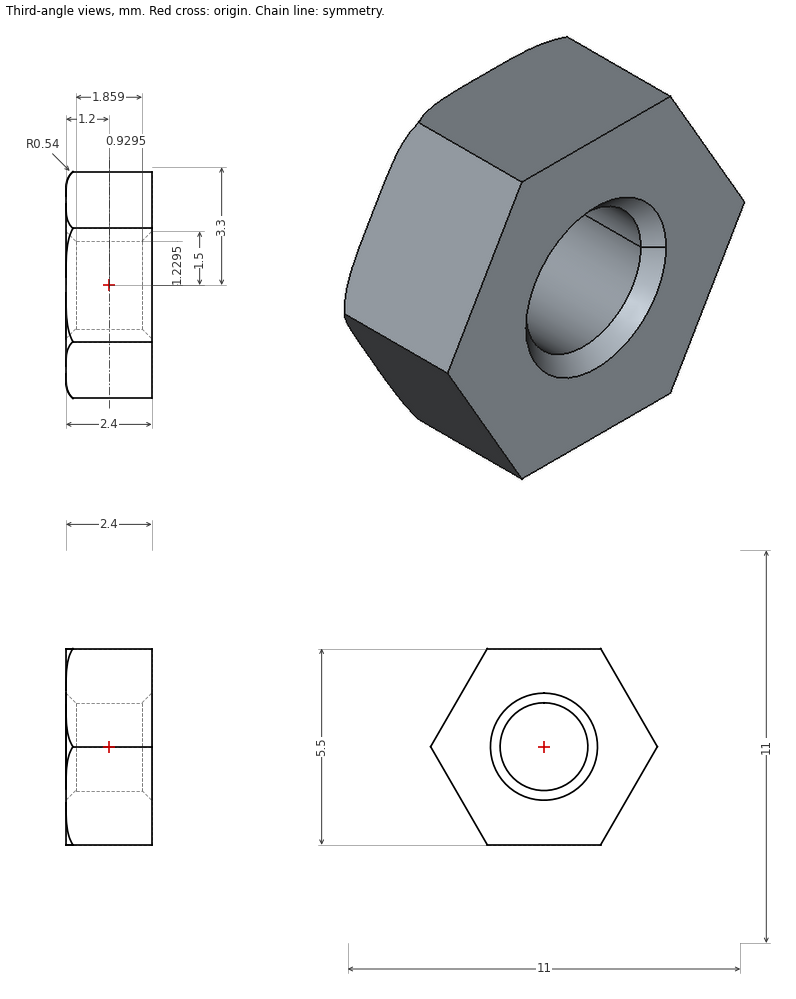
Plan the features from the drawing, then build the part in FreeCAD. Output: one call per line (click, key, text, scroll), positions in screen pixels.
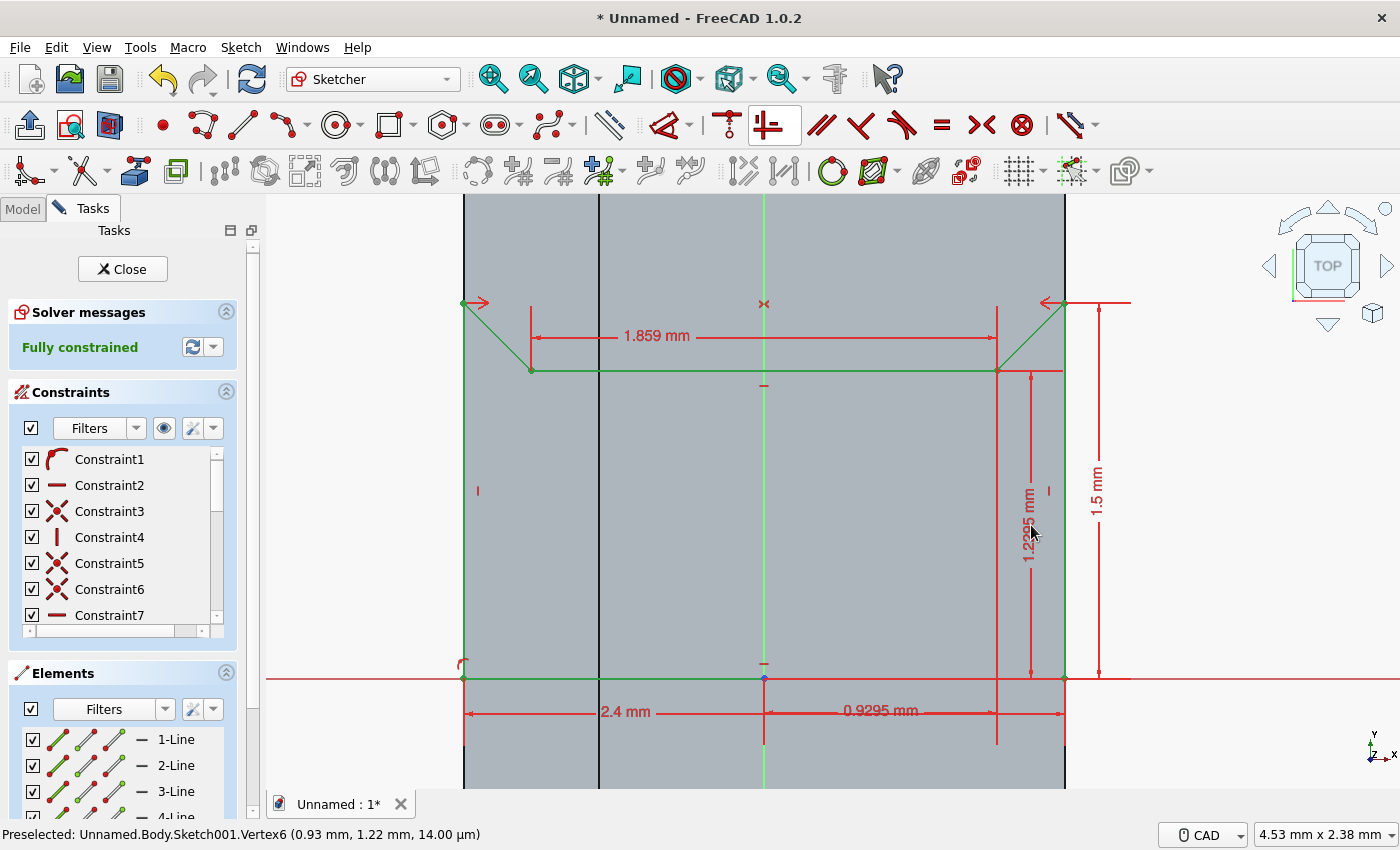
click(123, 269)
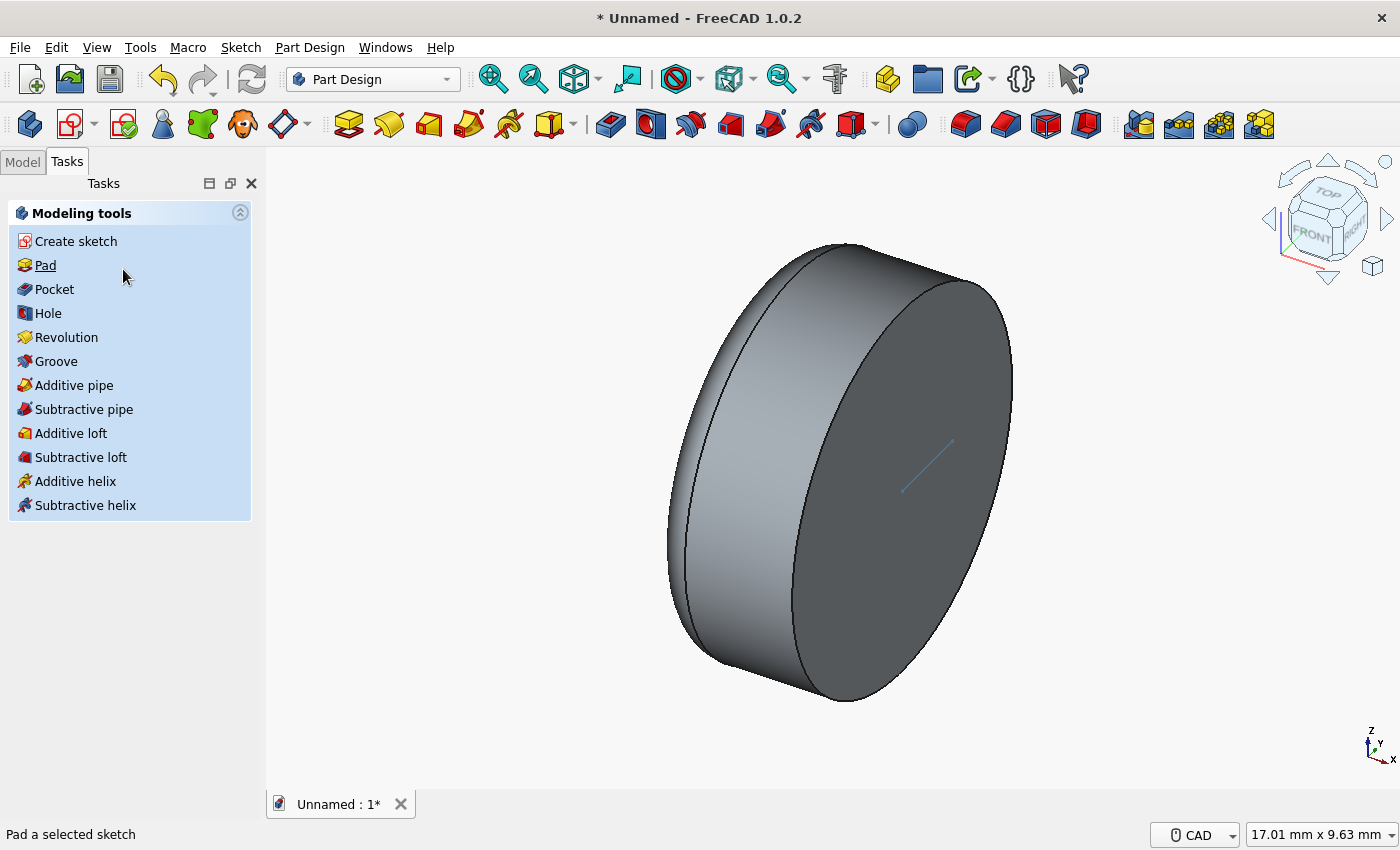
click(692, 124)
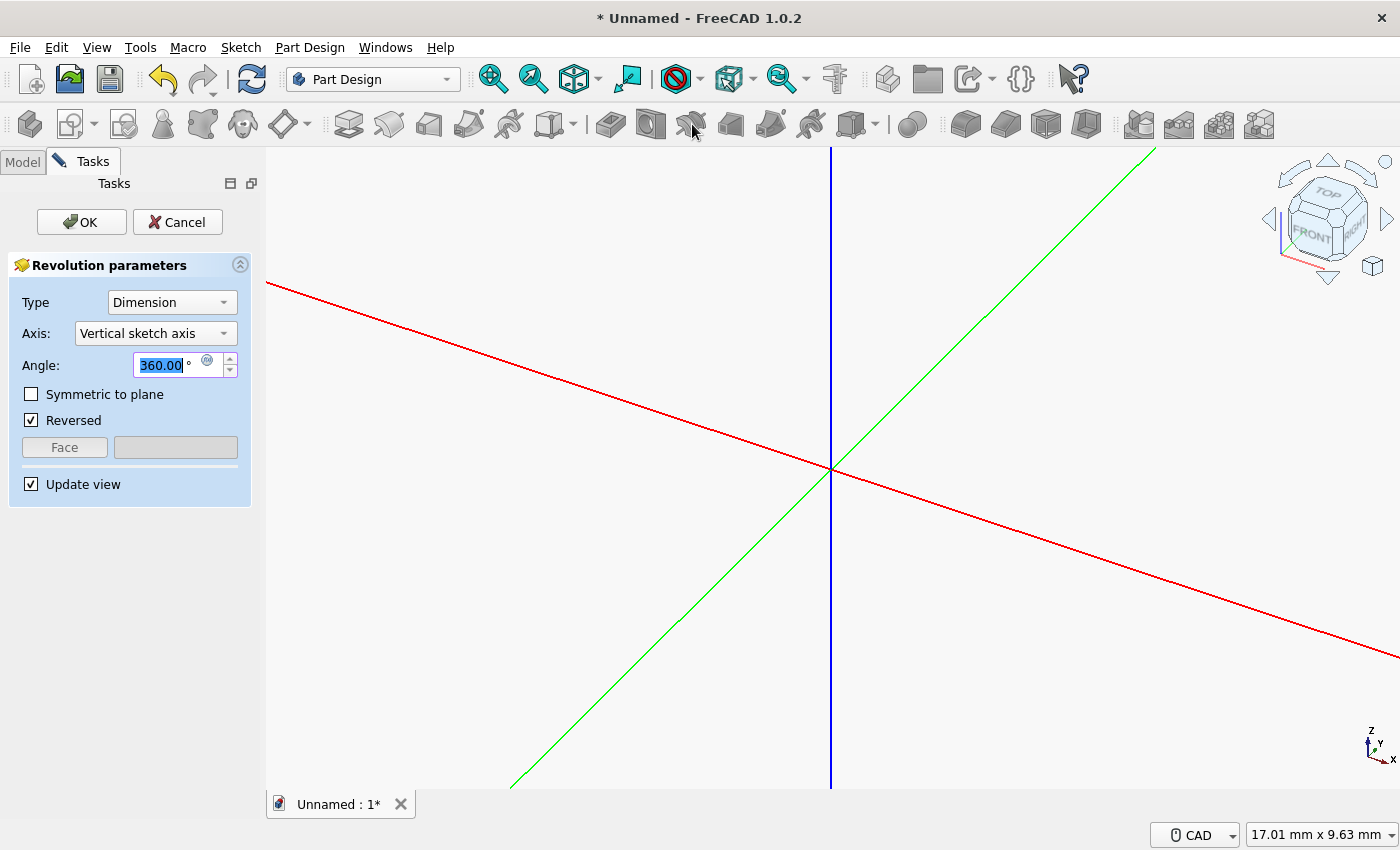
click(156, 334)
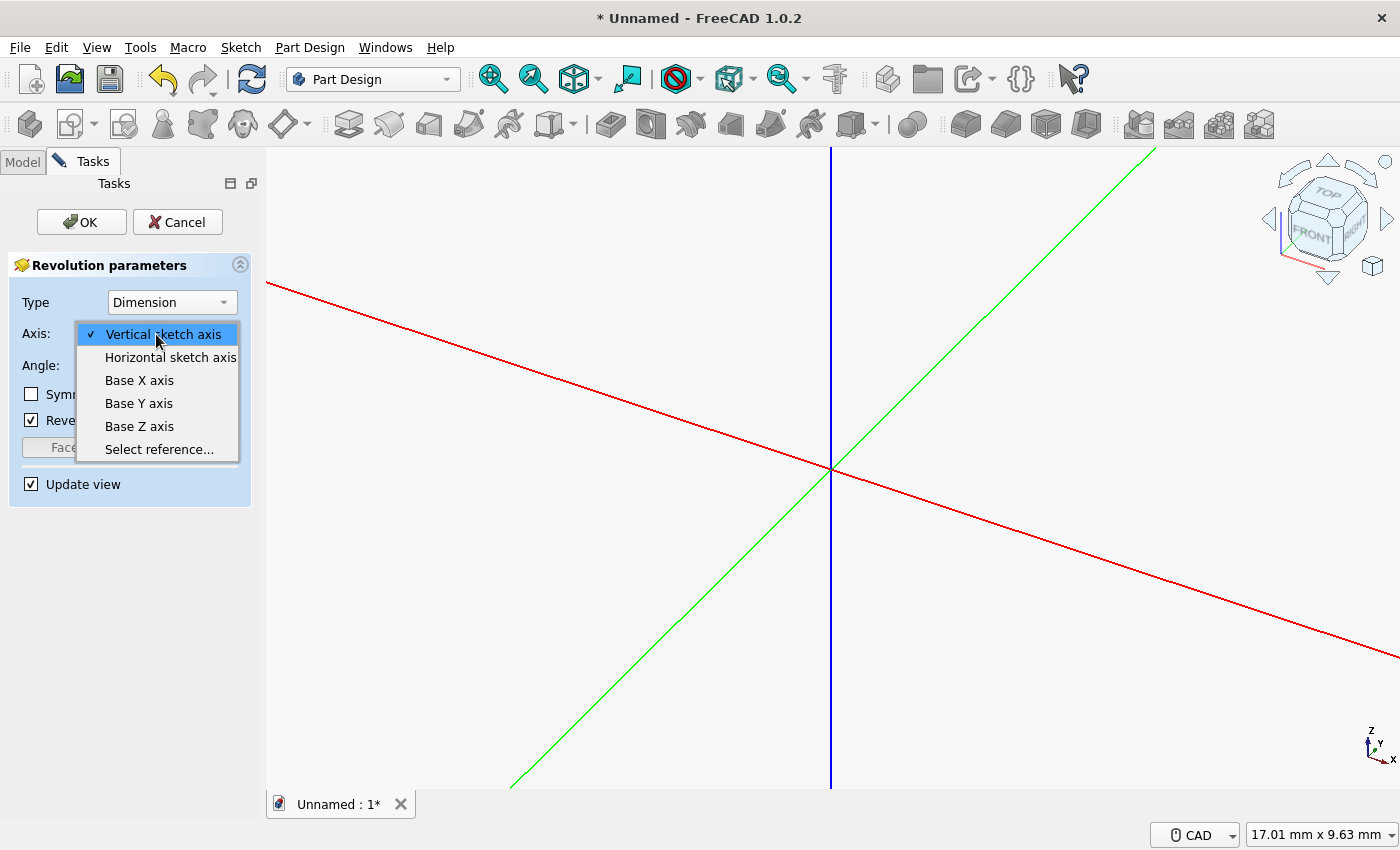
click(156, 358)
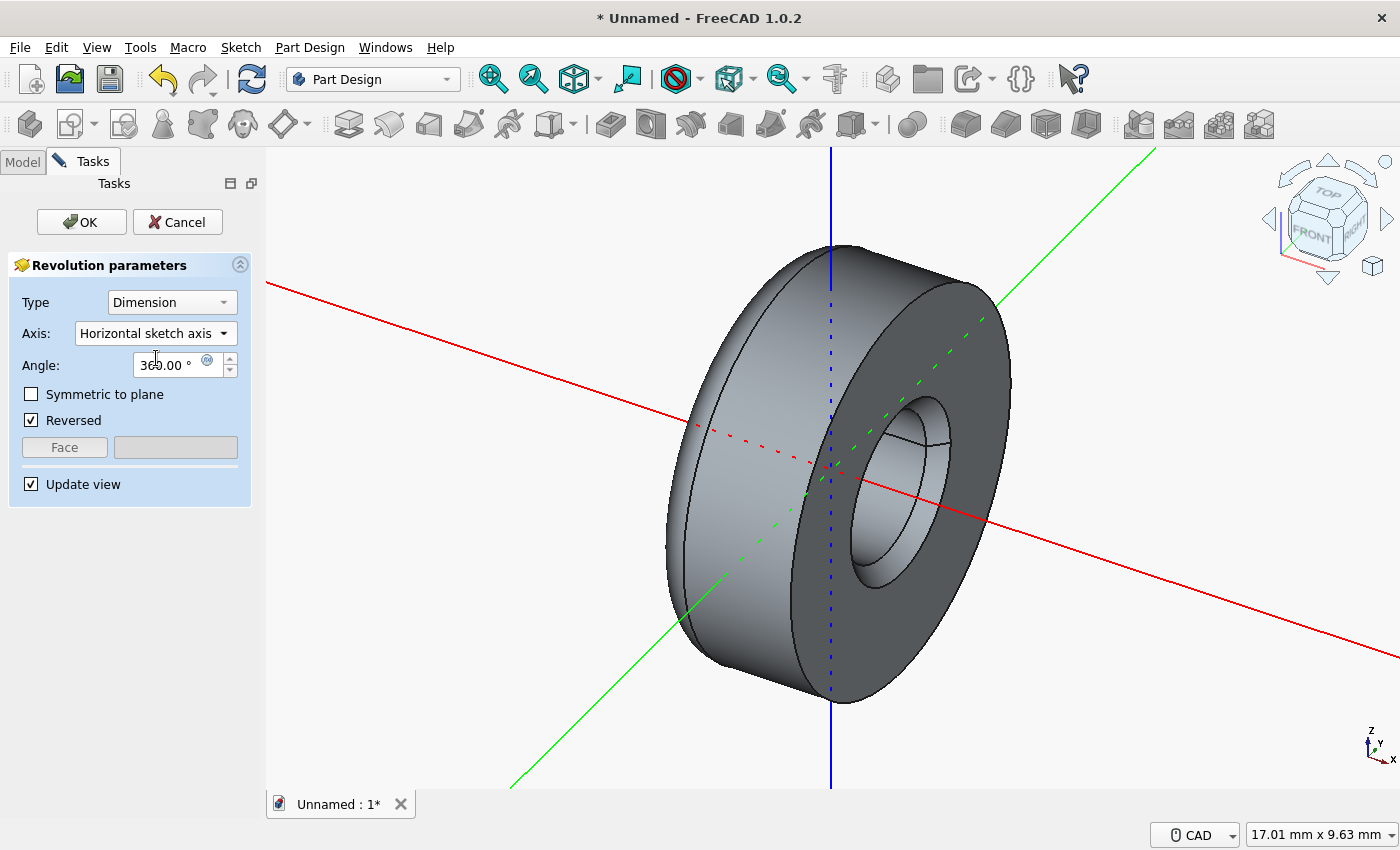
click(82, 222)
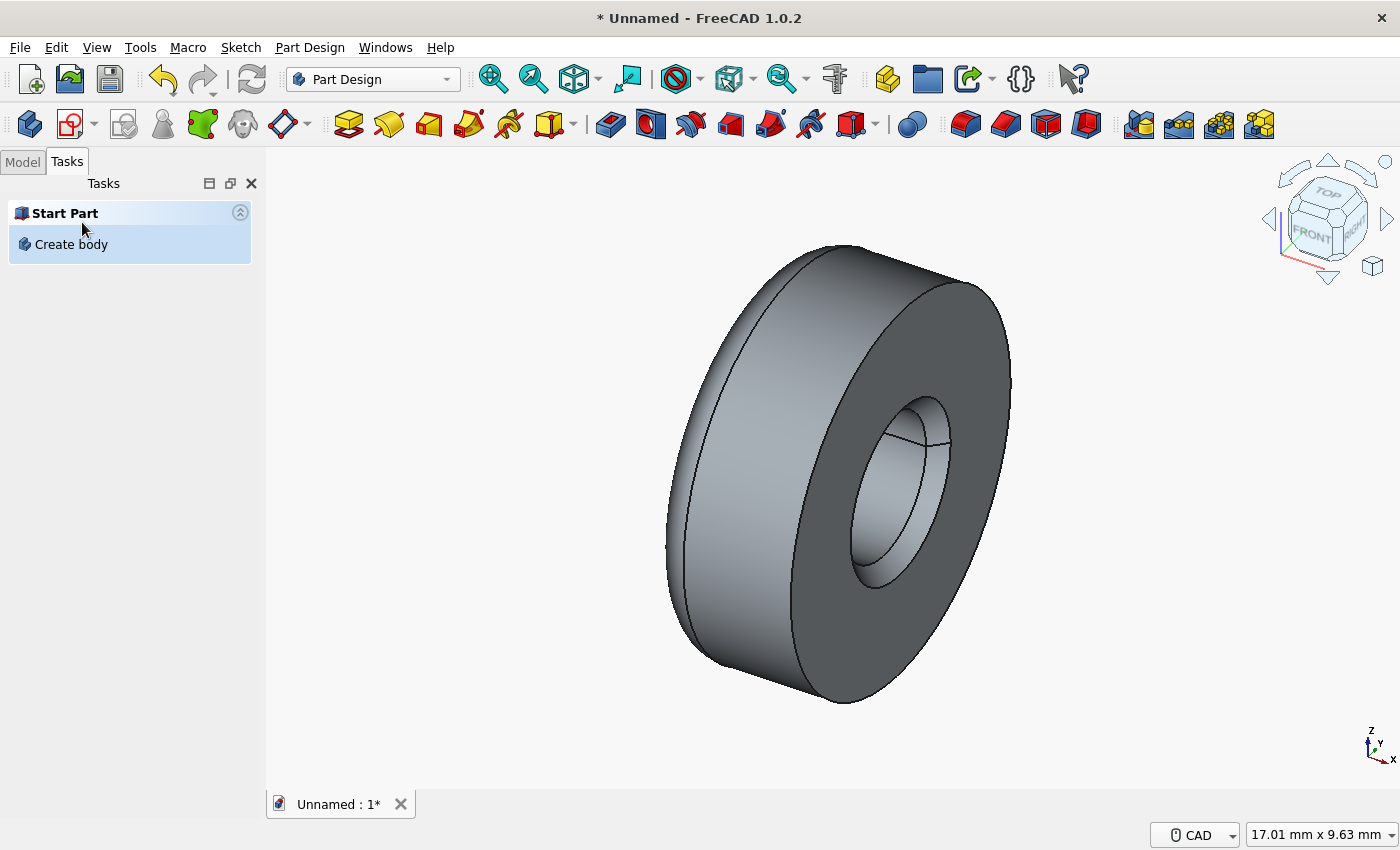
click(70, 124)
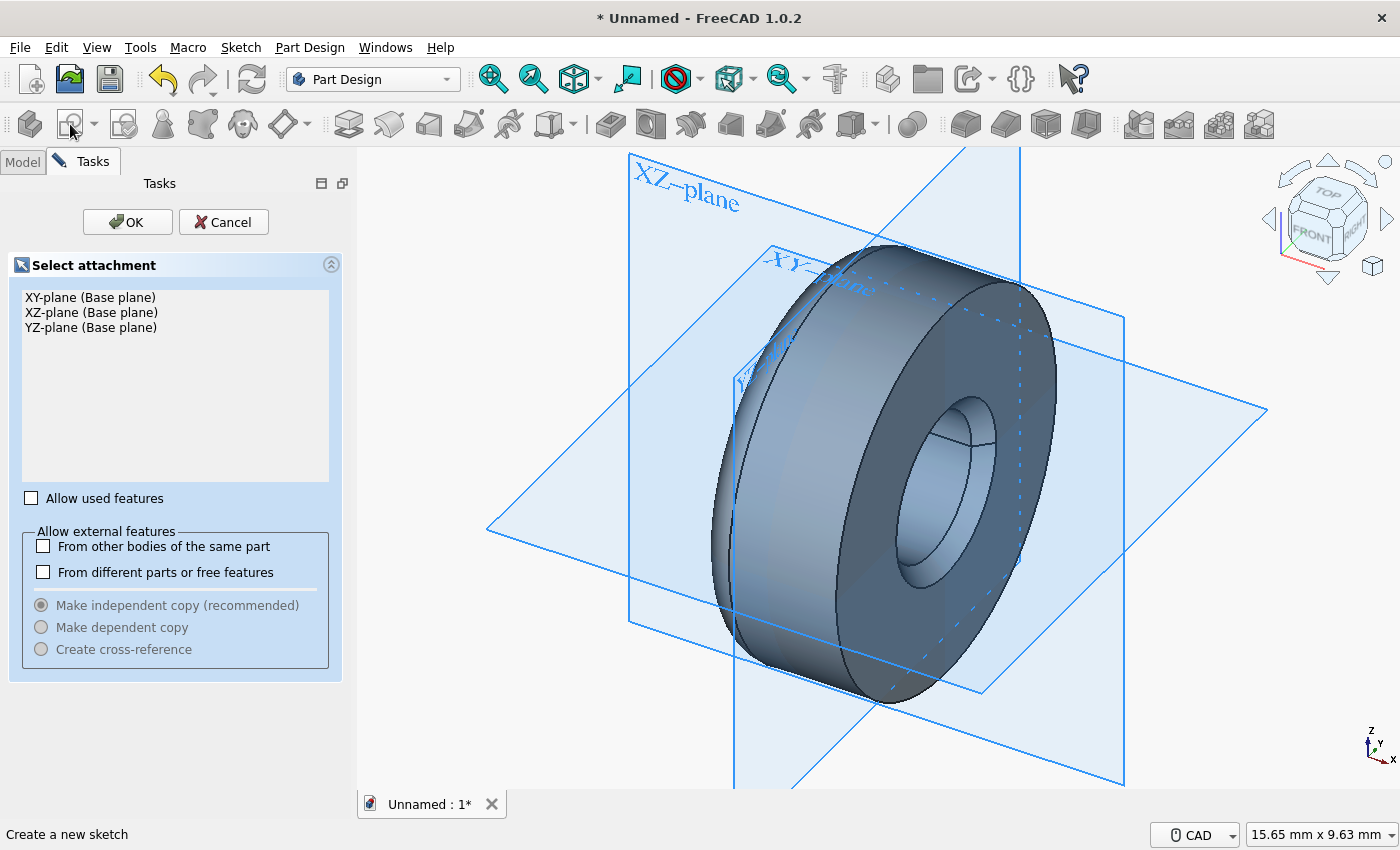
click(82, 328)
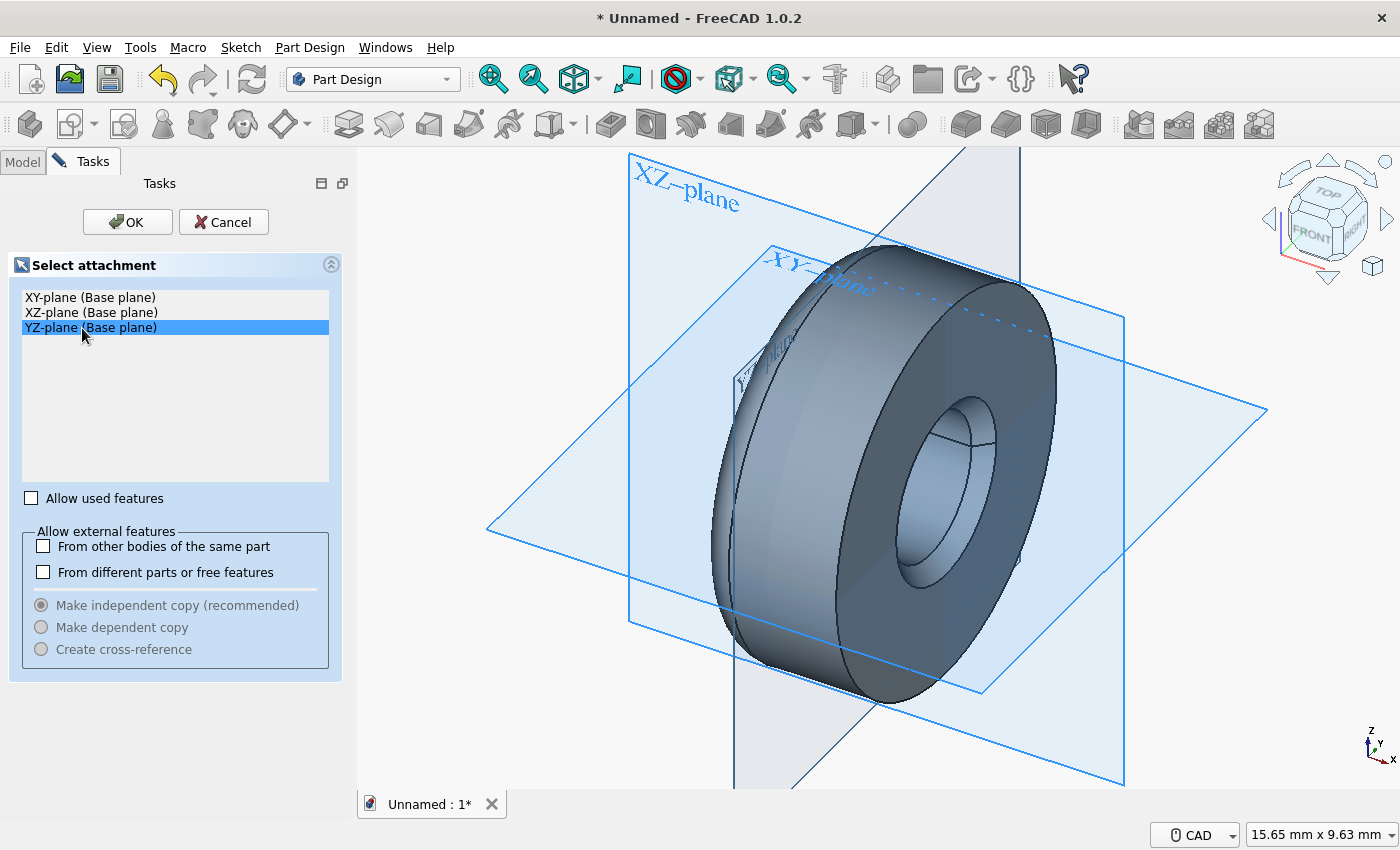
click(128, 222)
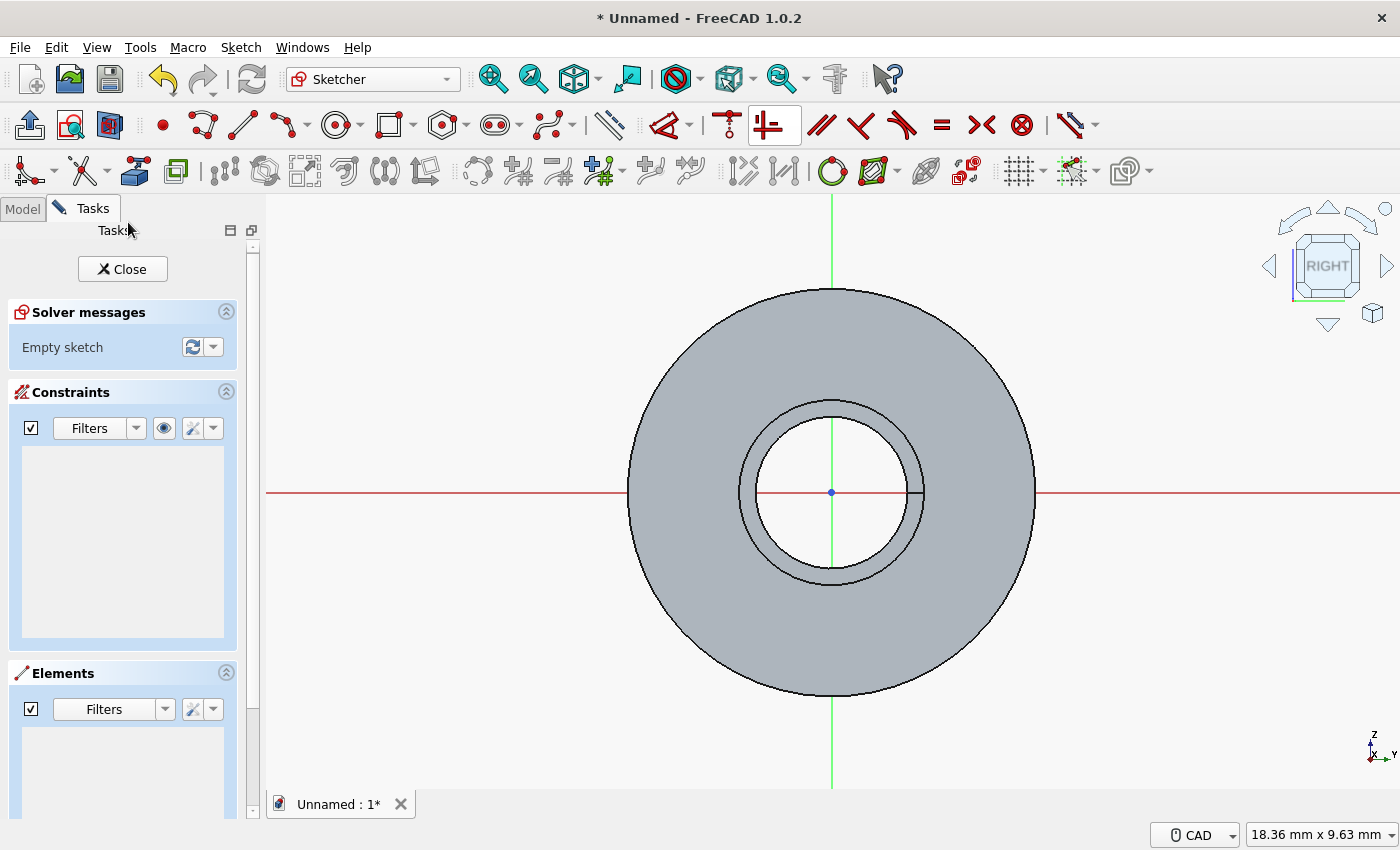
click(110, 126)